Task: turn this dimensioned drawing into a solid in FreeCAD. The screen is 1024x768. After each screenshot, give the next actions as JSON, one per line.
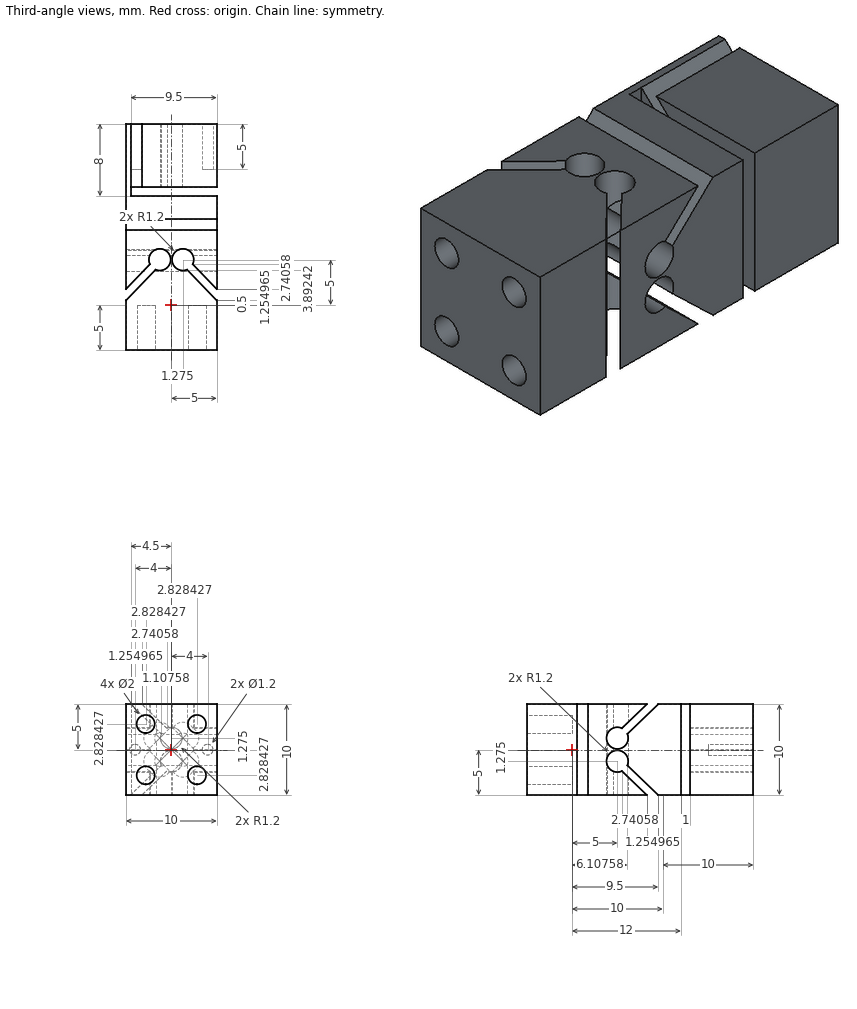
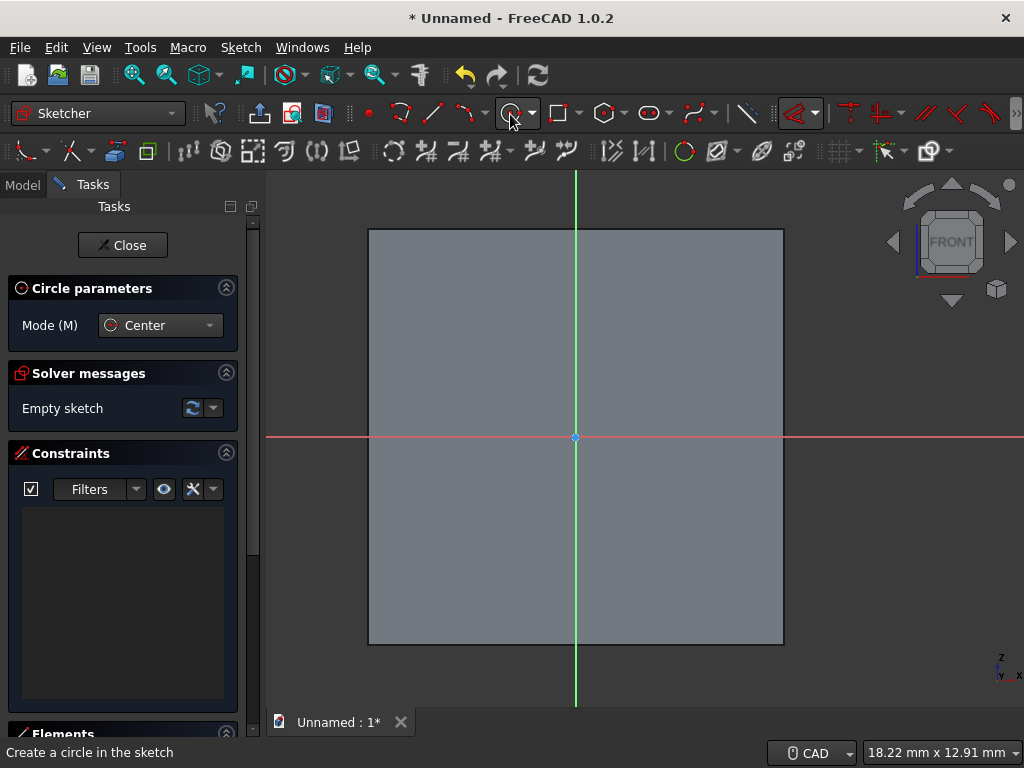
{"action": "left_click", "coordinate": [458, 320]}
{"action": "left_click", "coordinate": [487, 290]}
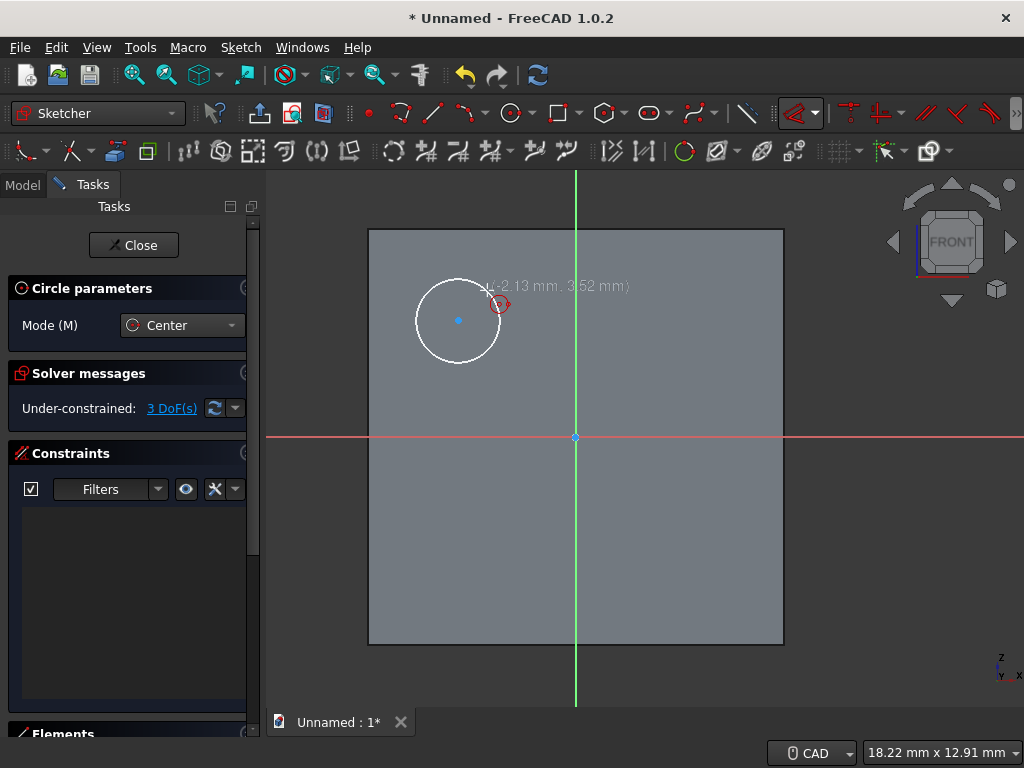
{"action": "left_click", "coordinate": [693, 320]}
{"action": "left_click", "coordinate": [723, 290]}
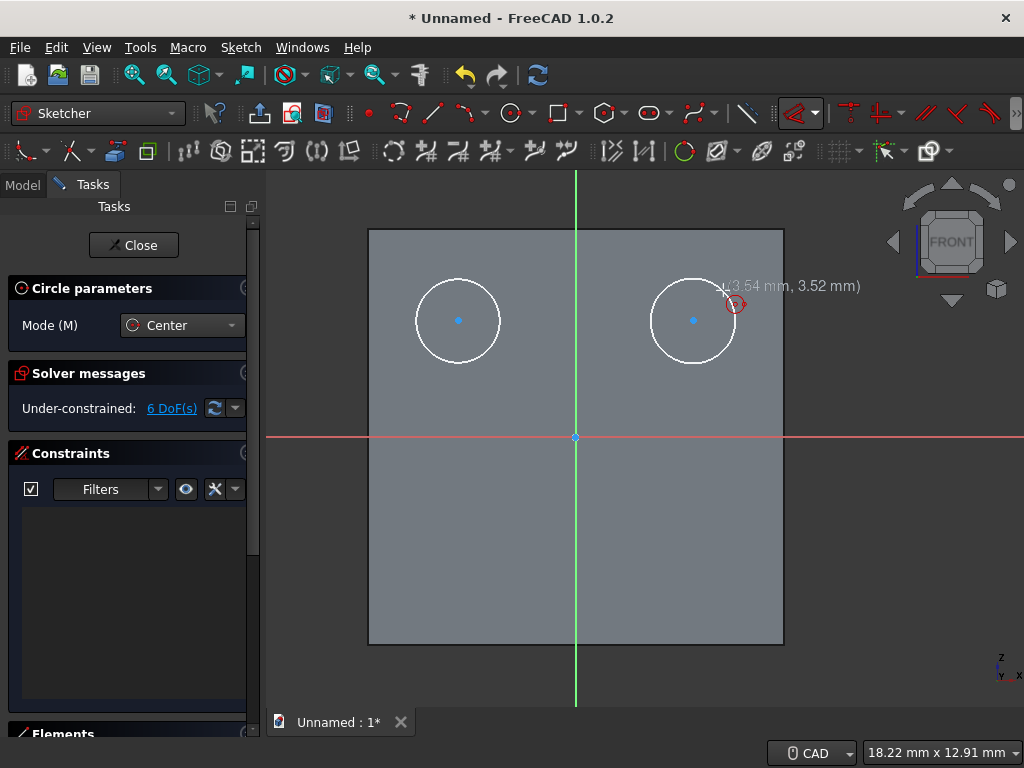
{"action": "left_click", "coordinate": [693, 555]}
{"action": "left_click", "coordinate": [723, 526]}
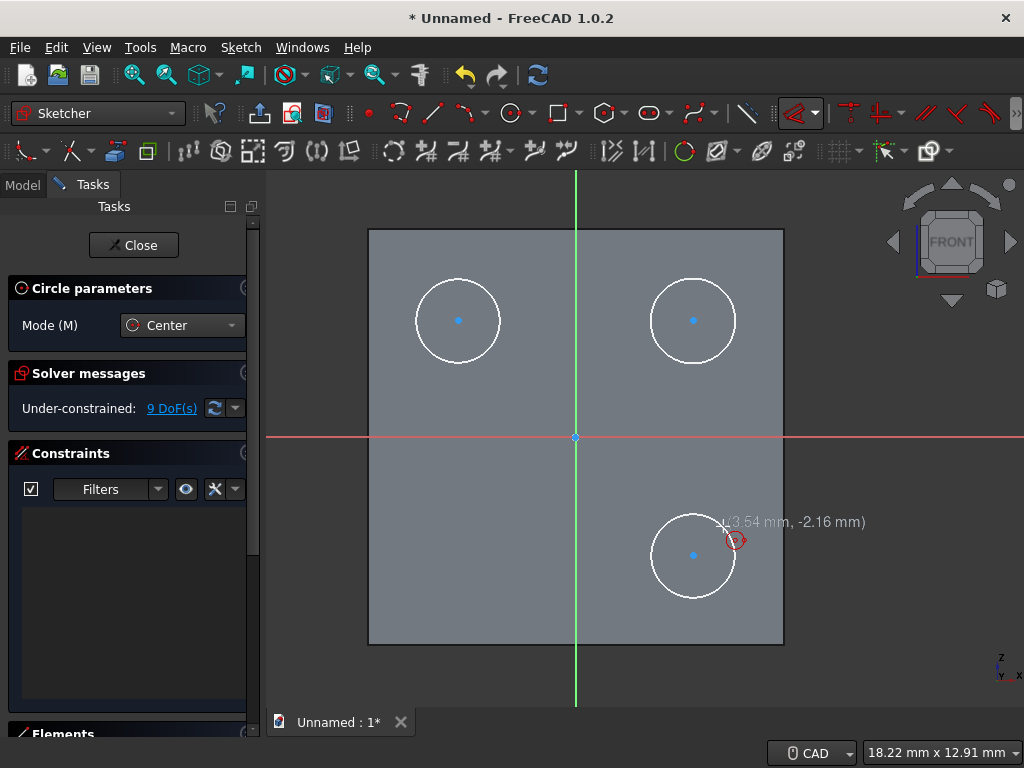
{"action": "left_click", "coordinate": [458, 555]}
{"action": "left_click", "coordinate": [487, 526]}
{"action": "key", "text": "Escape"}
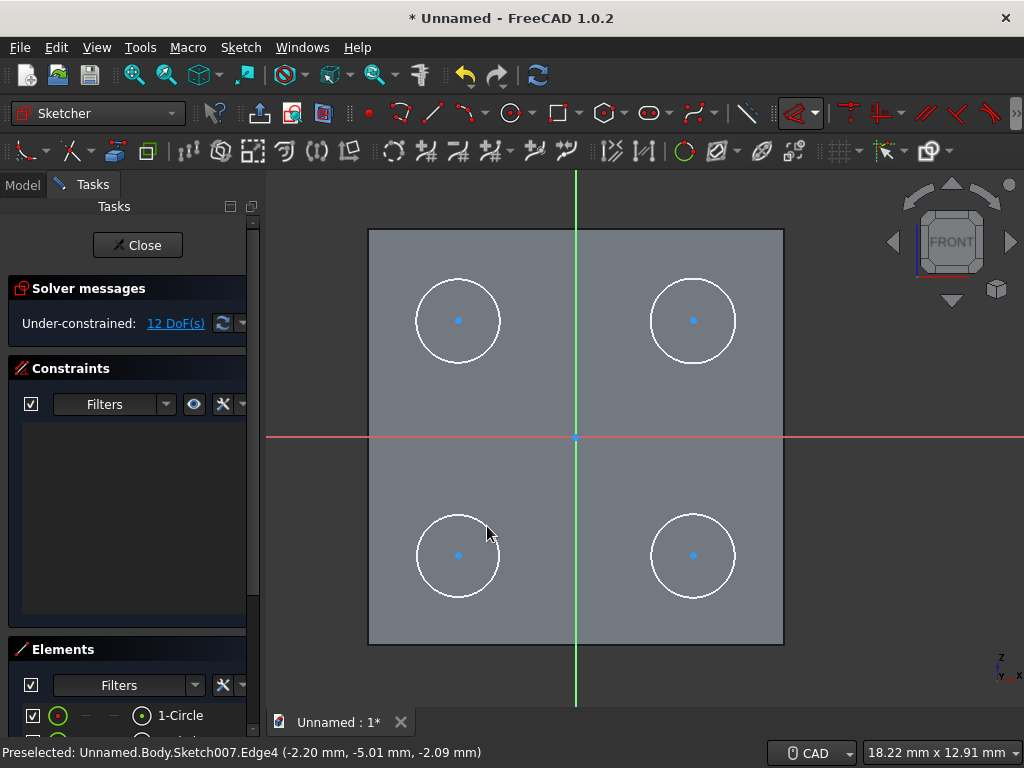
{"action": "left_click", "coordinate": [487, 291]}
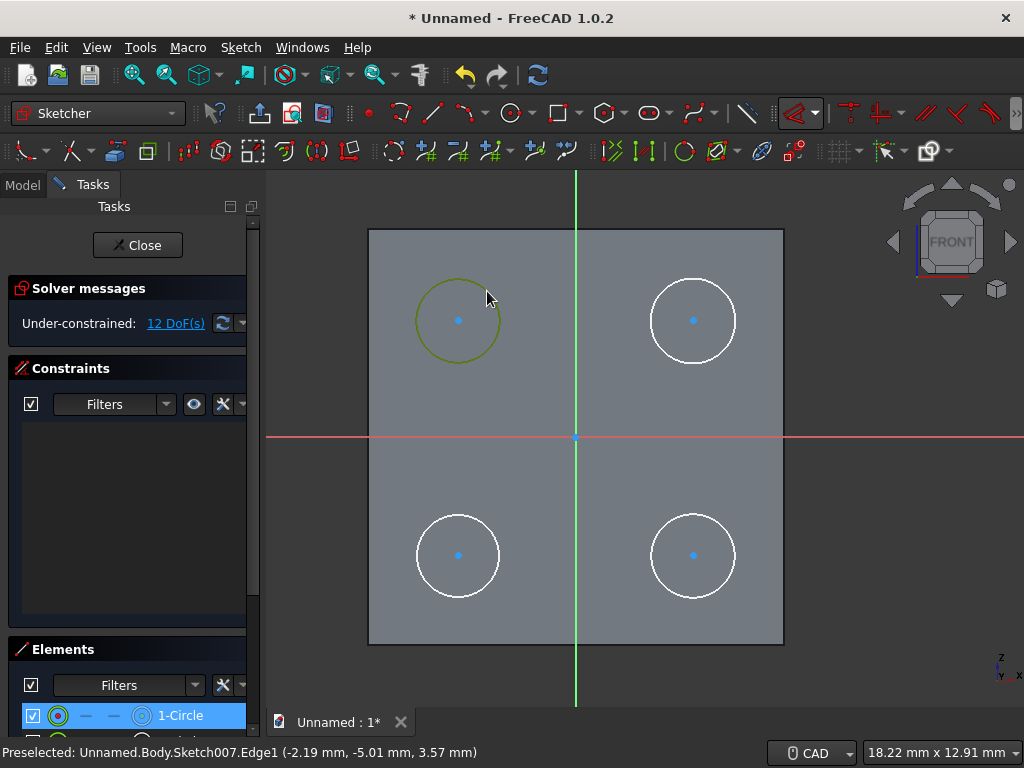
{"action": "left_click", "coordinate": [723, 291]}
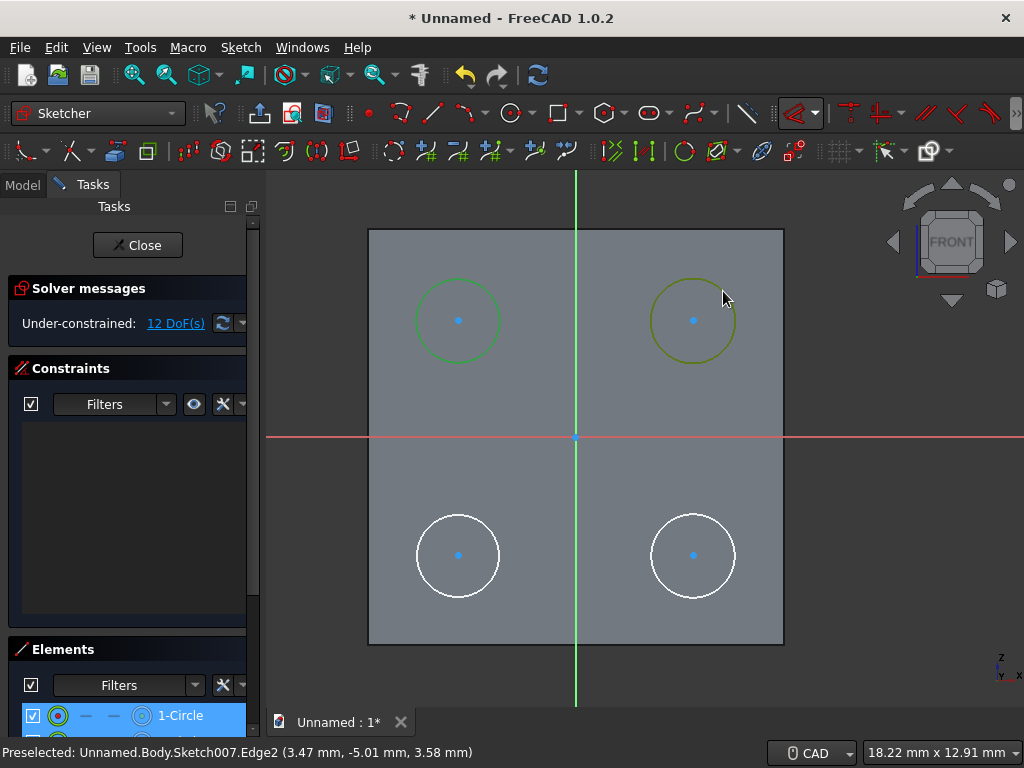
{"action": "left_click", "coordinate": [722, 526]}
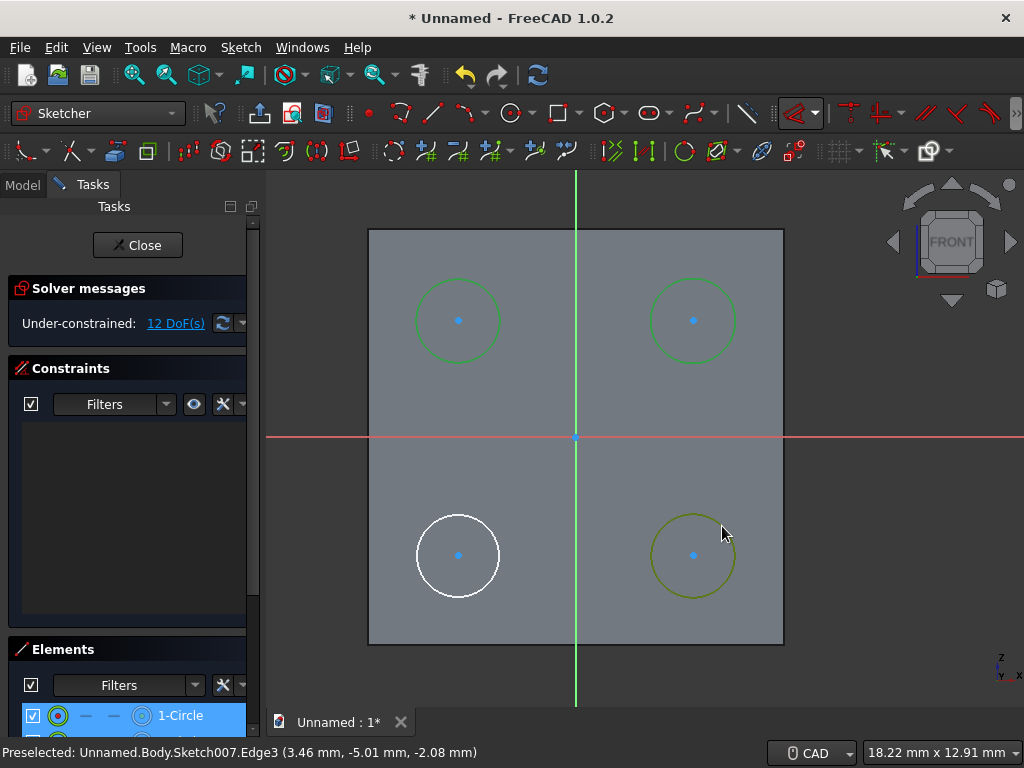
{"action": "left_click", "coordinate": [487, 527]}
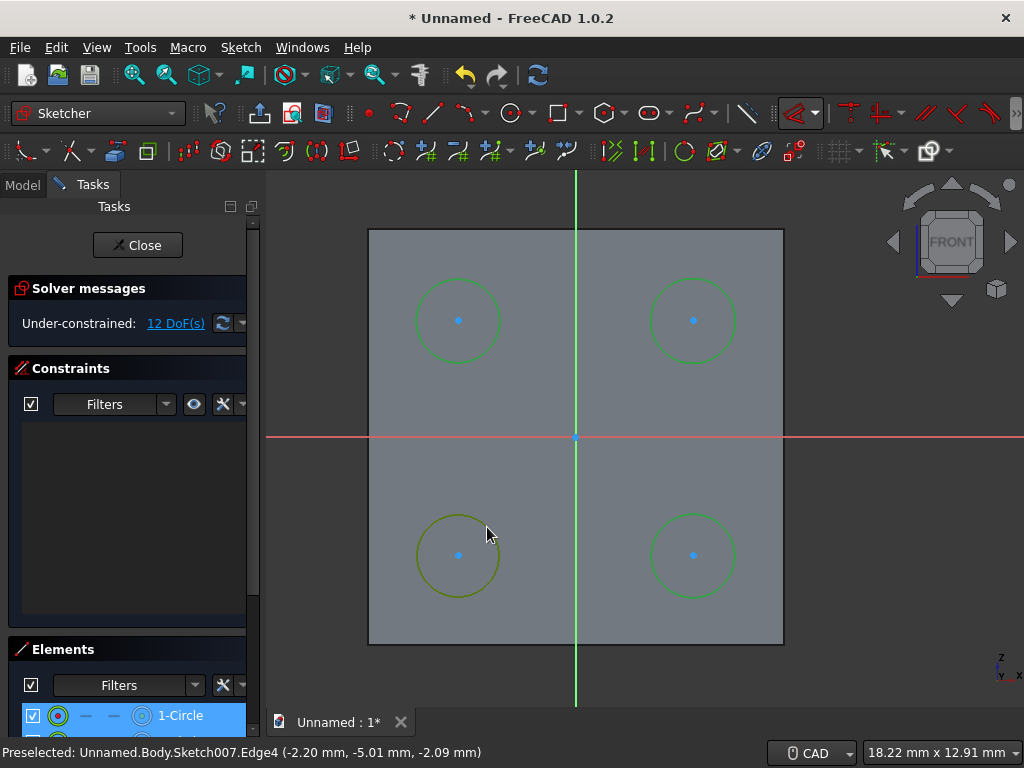
{"action": "key", "text": "e"}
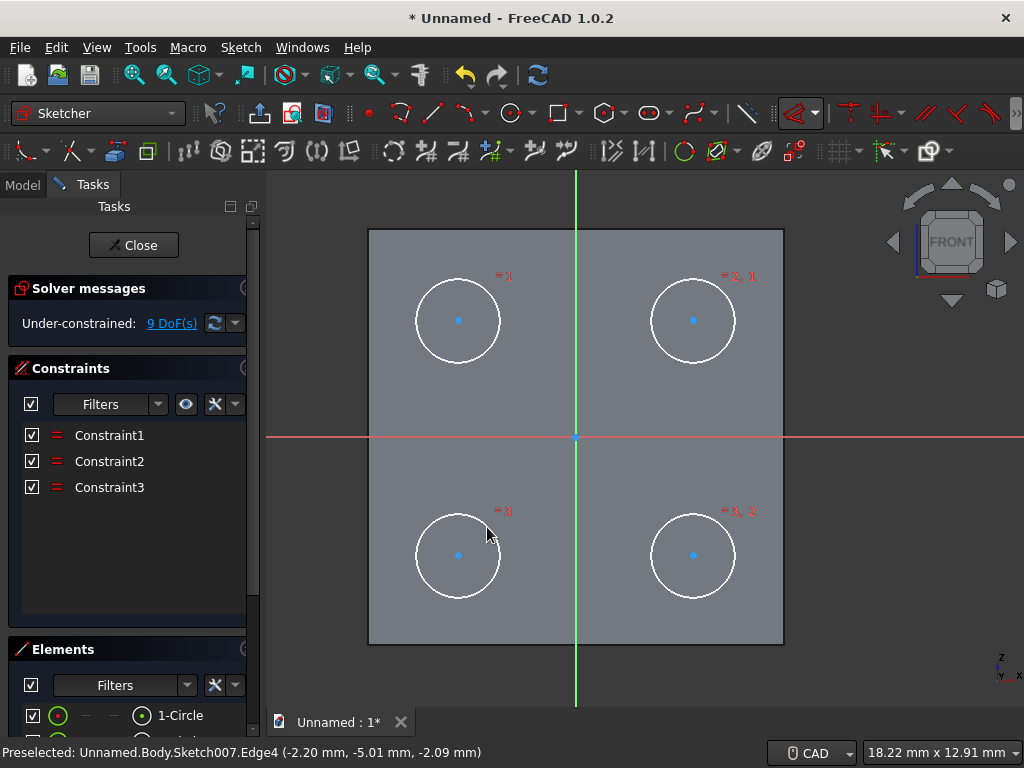
{"action": "left_click", "coordinate": [458, 321]}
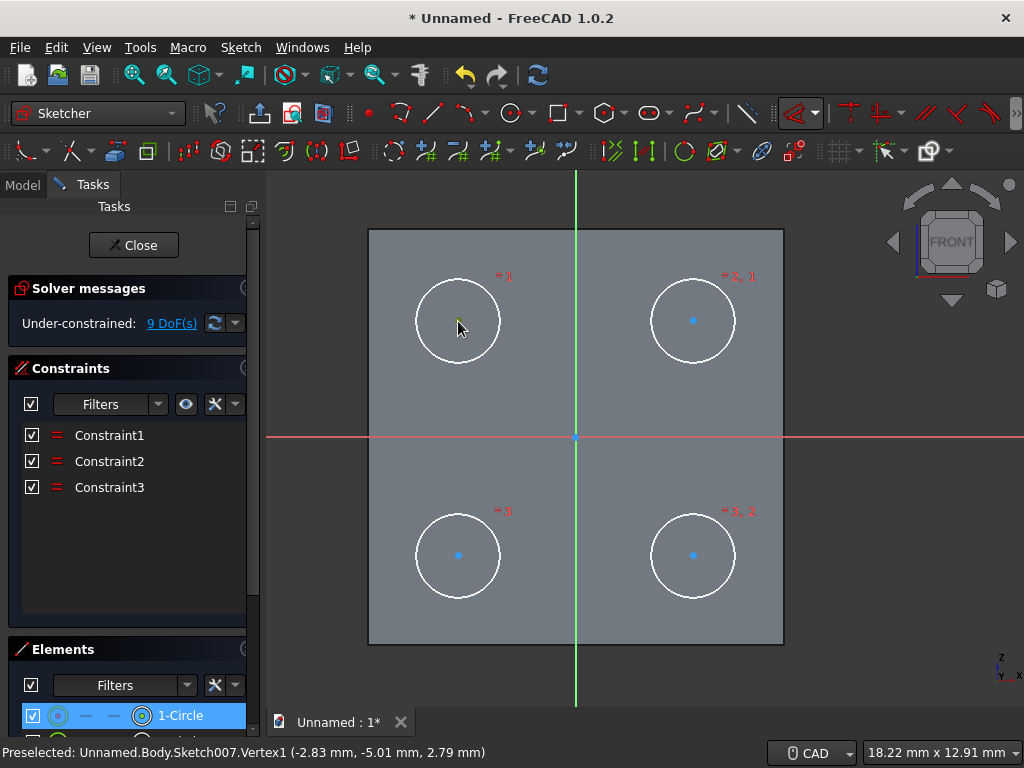
{"action": "left_click", "coordinate": [693, 321]}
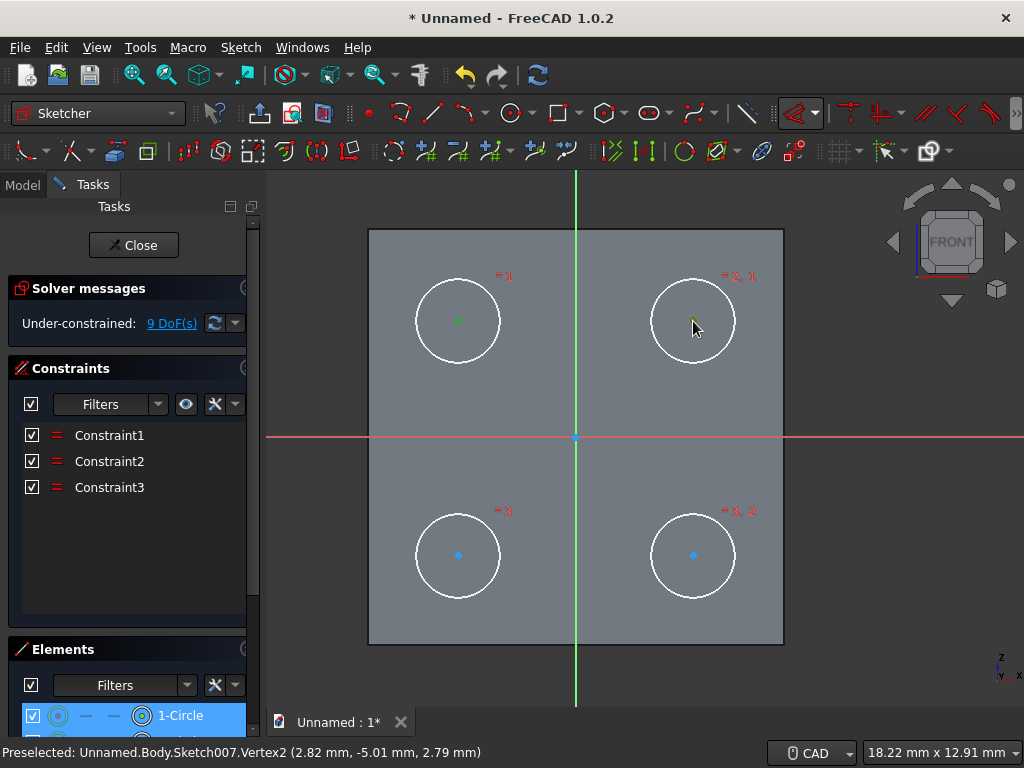
{"action": "left_click", "coordinate": [904, 114]}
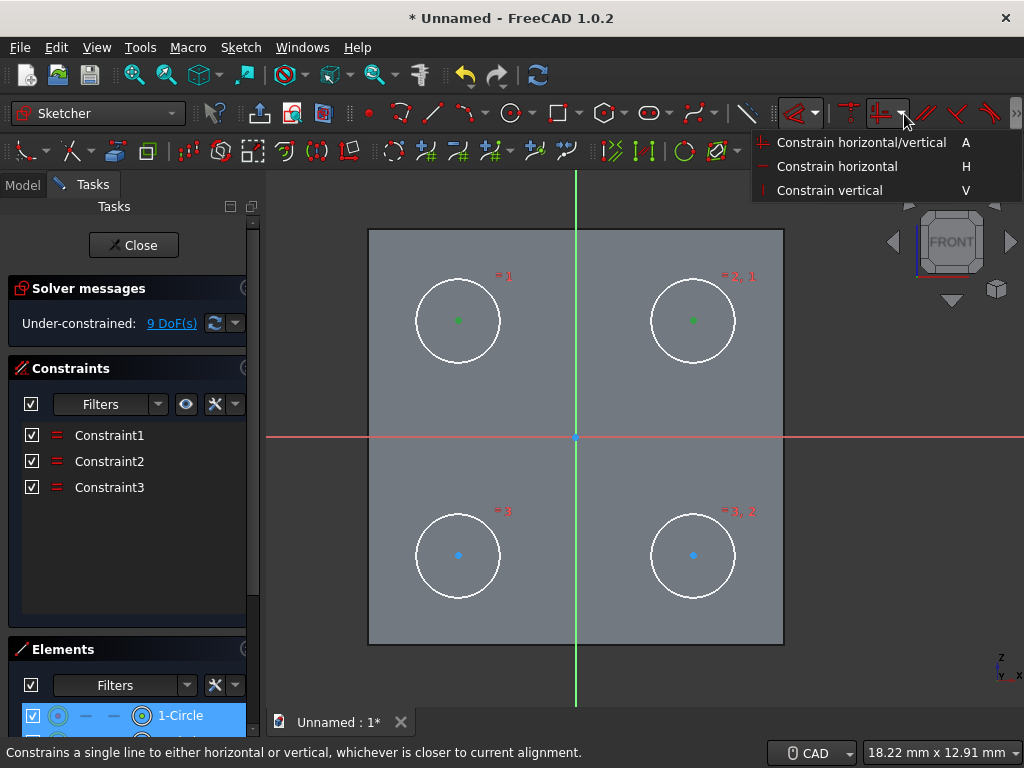
{"action": "left_click", "coordinate": [887, 166]}